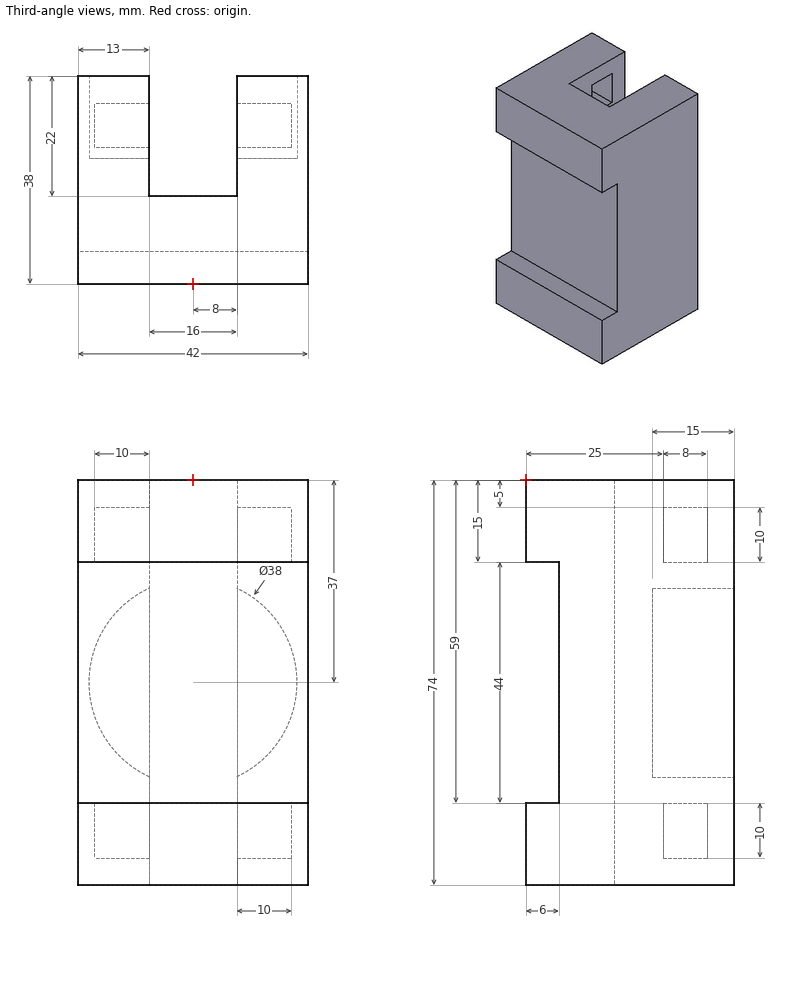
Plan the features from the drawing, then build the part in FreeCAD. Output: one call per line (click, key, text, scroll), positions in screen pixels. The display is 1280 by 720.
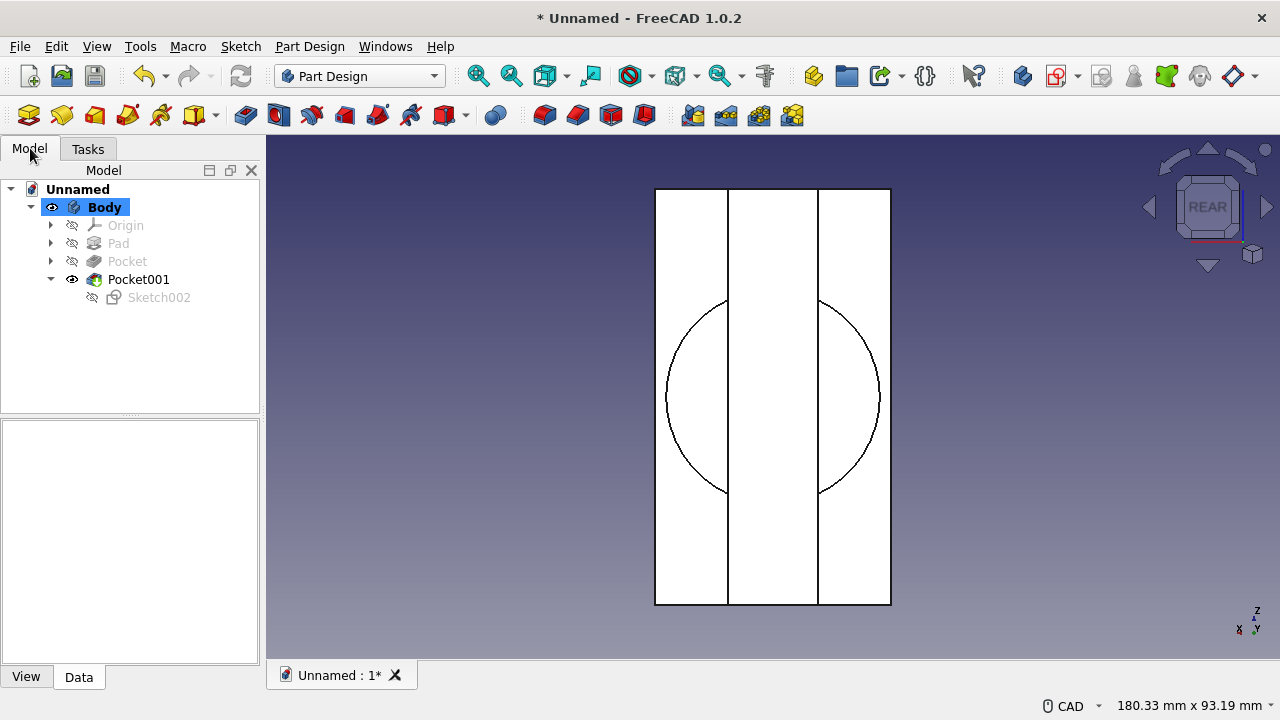
click(51, 225)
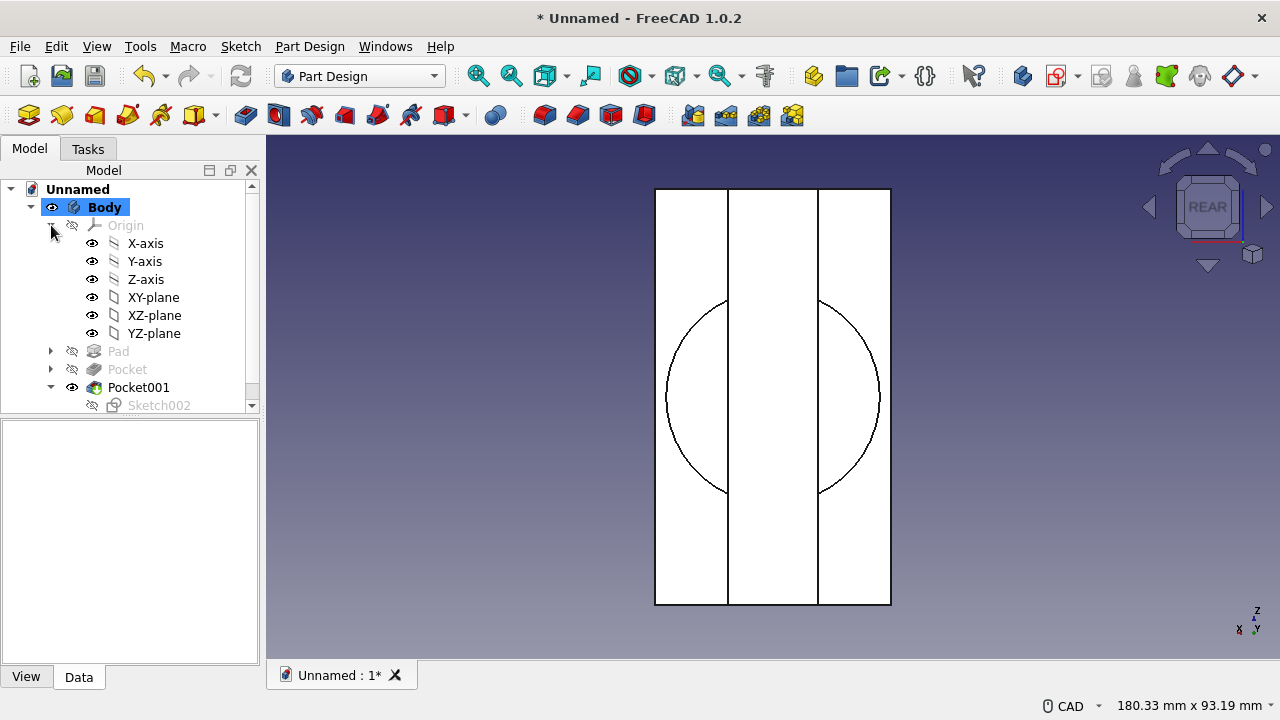
click(137, 333)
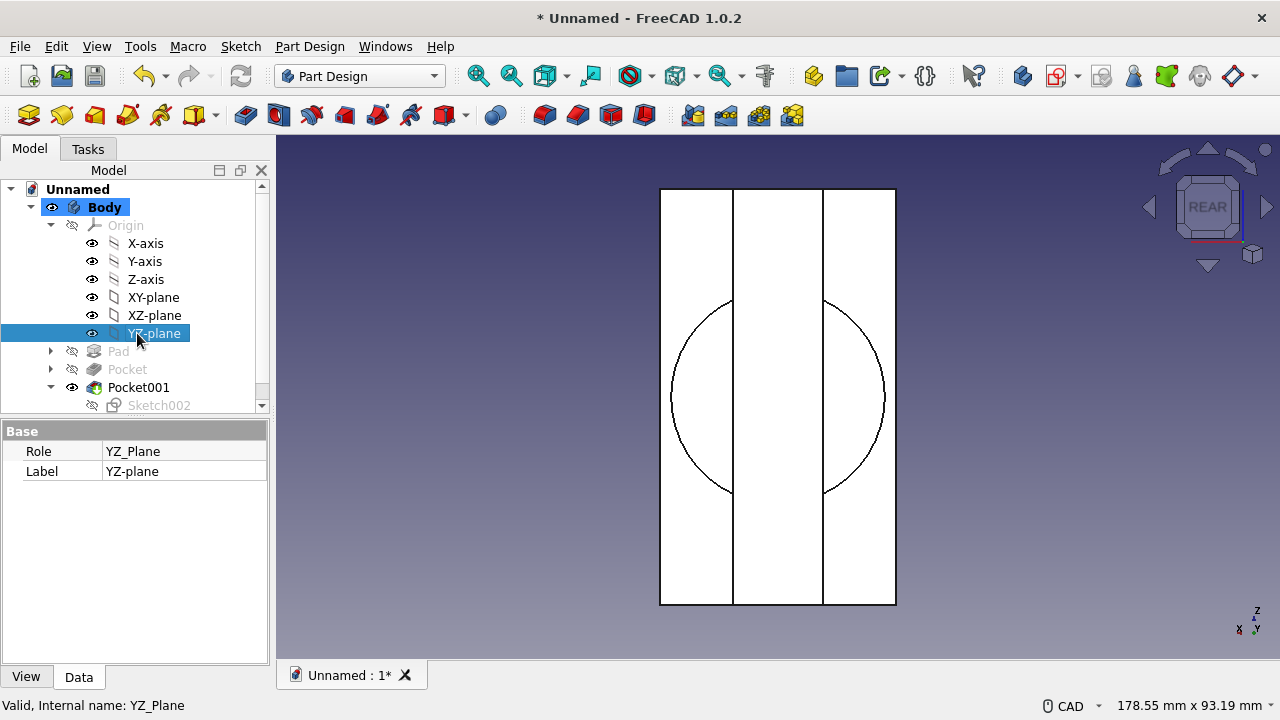
click(1232, 76)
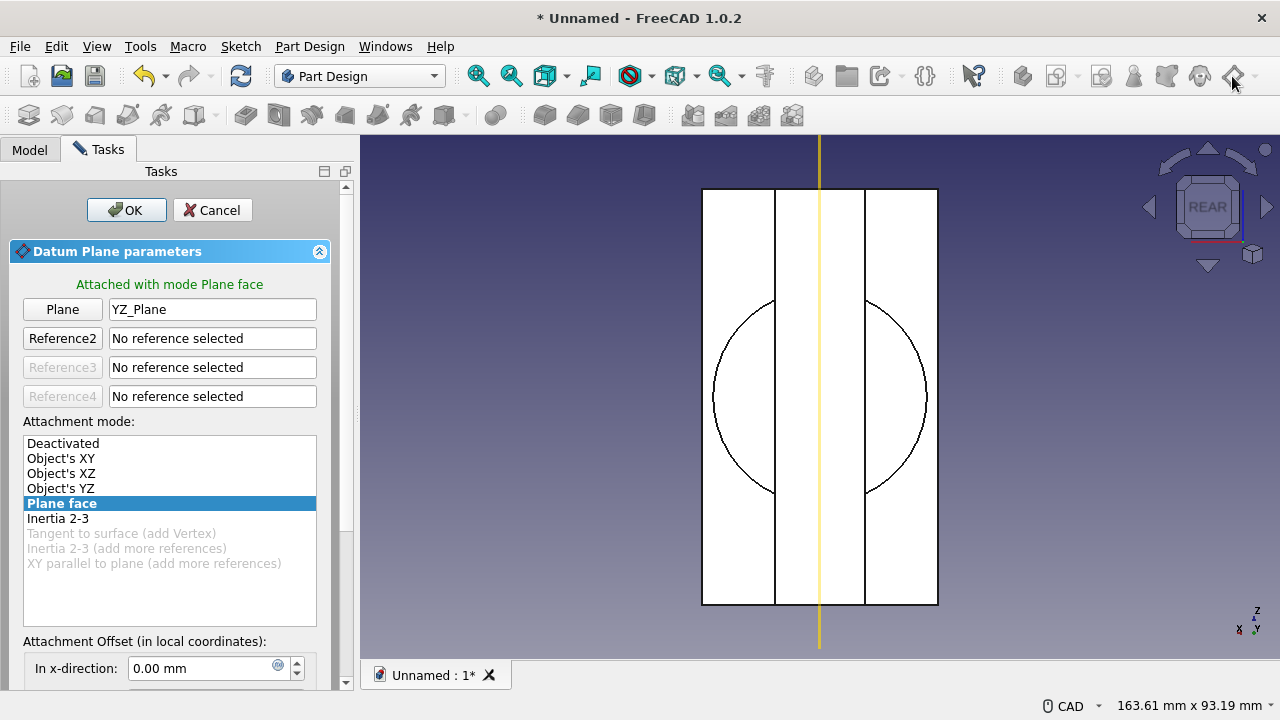
scroll(346, 436, down, 2)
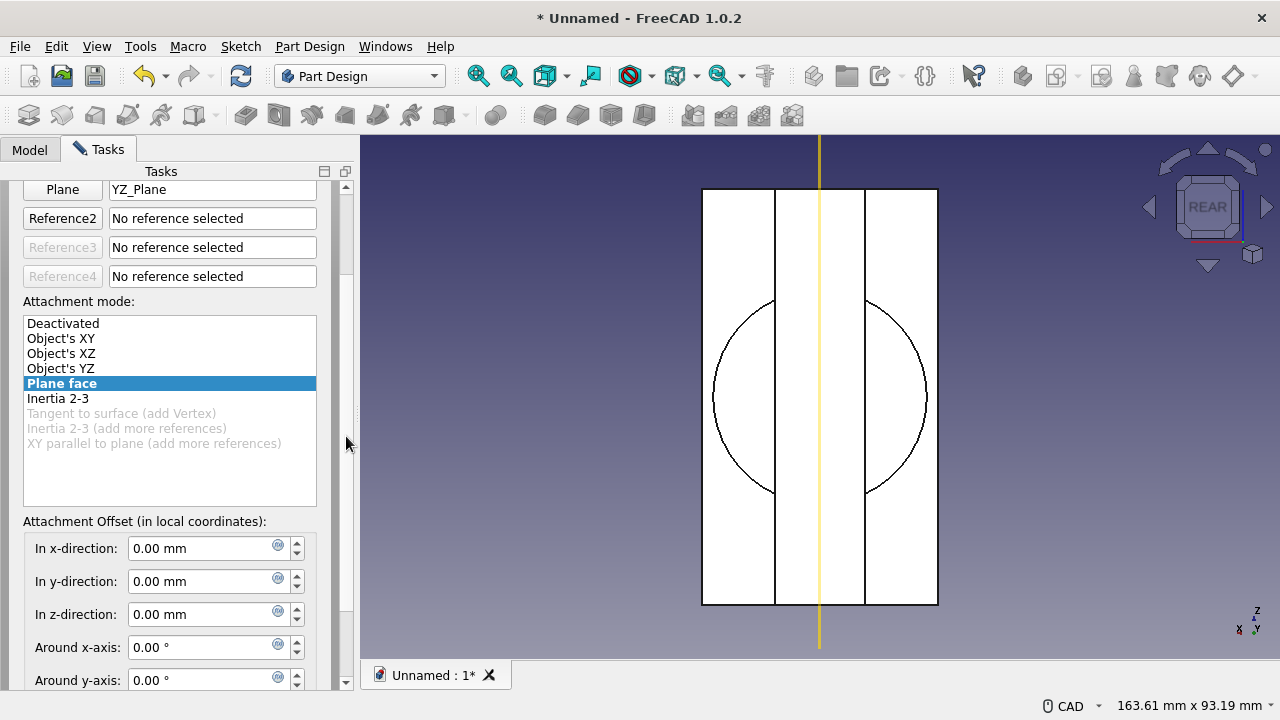
triple_click(210, 614)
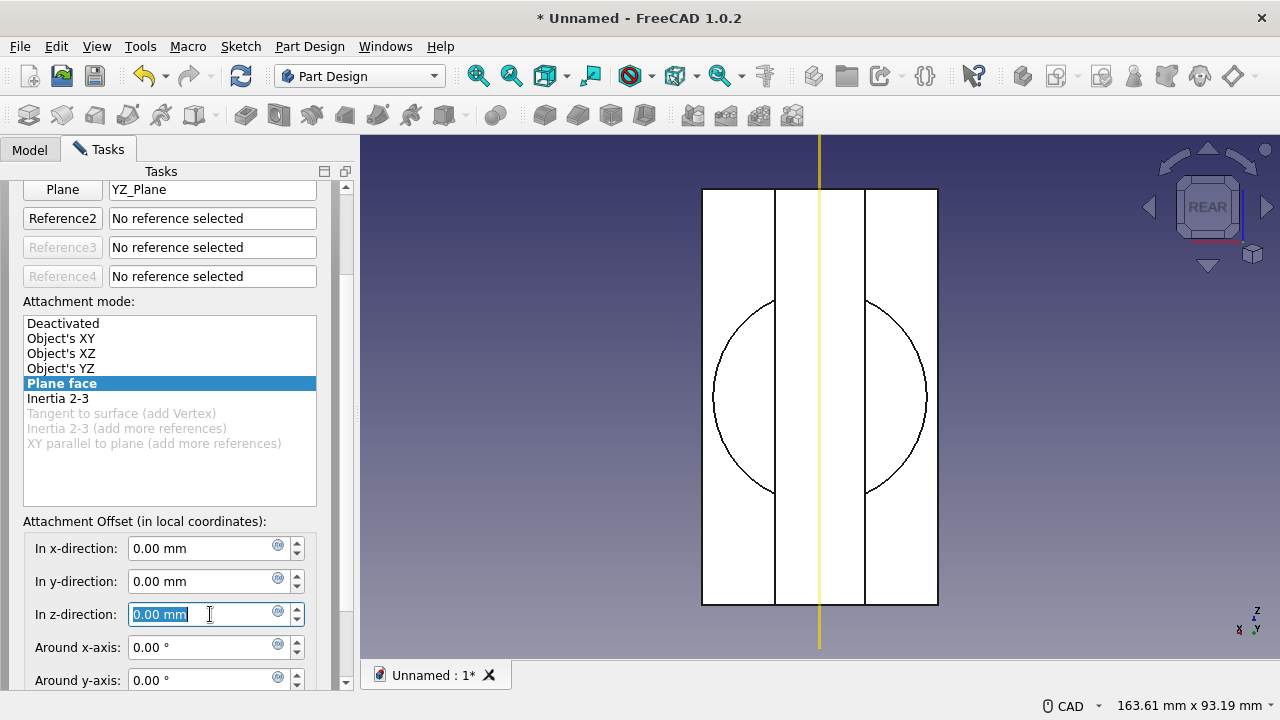
text(-8)
key(Tab)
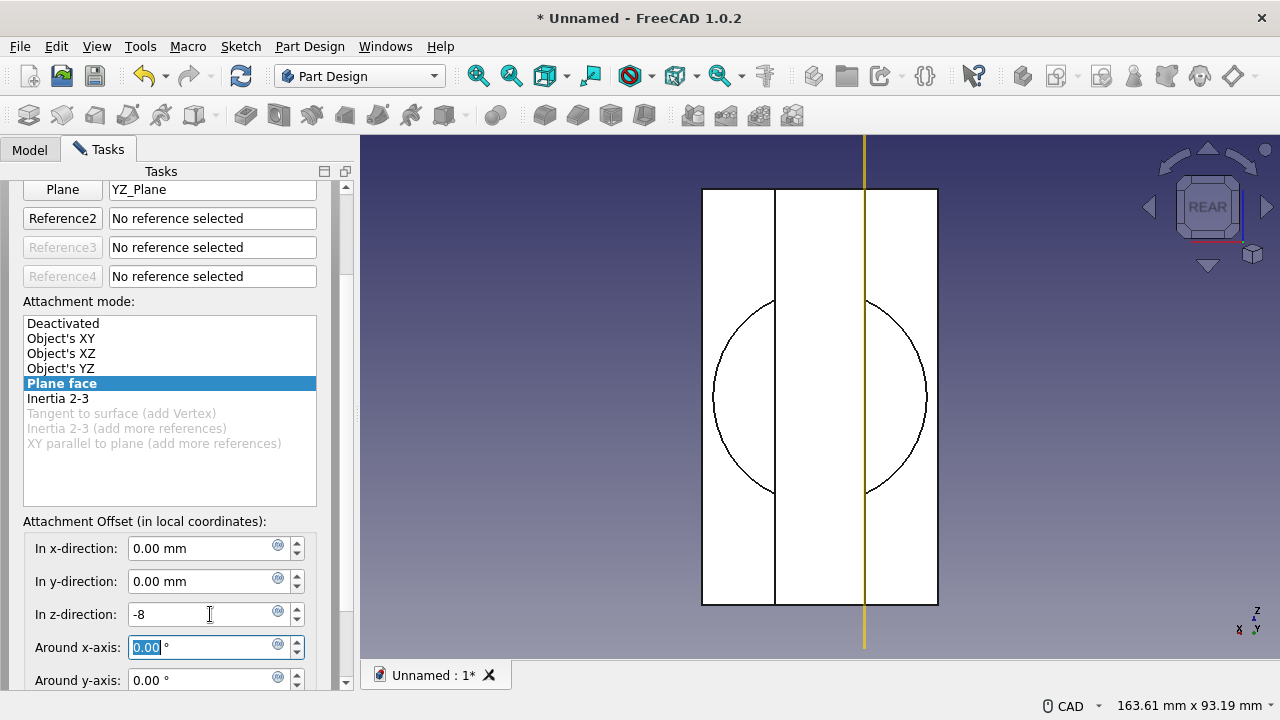
scroll(346, 436, up, 3)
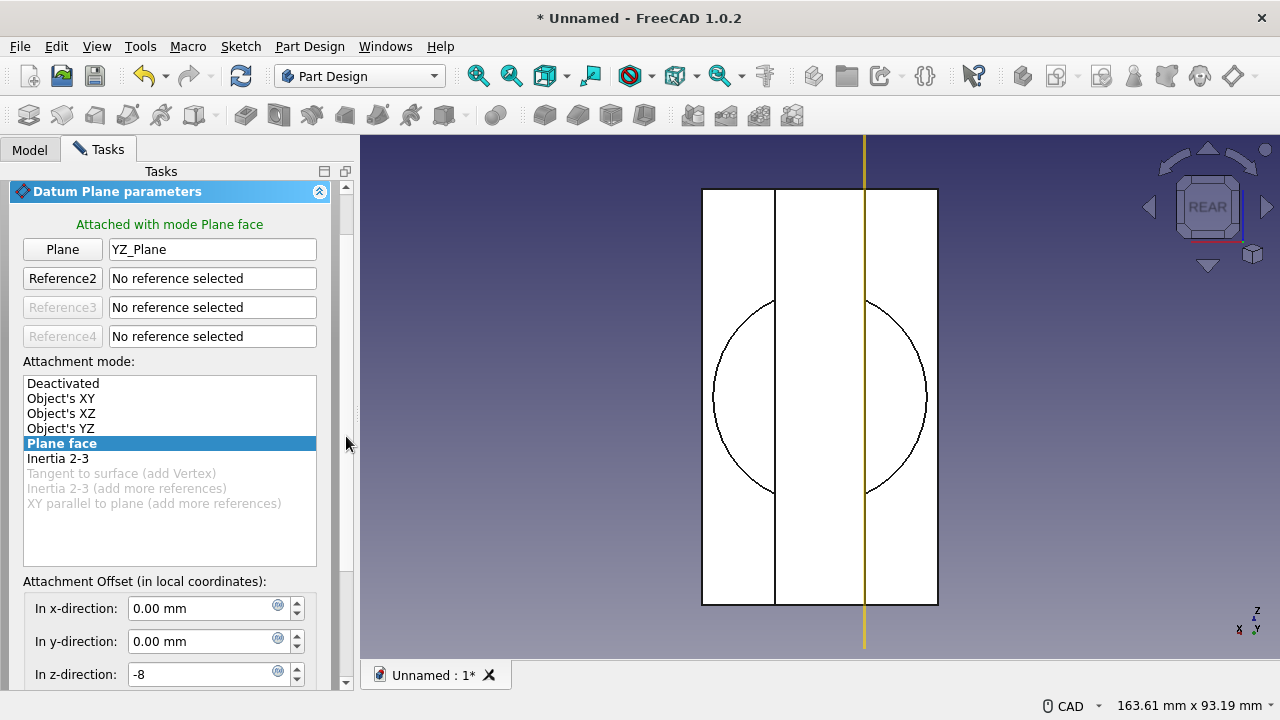
click(127, 210)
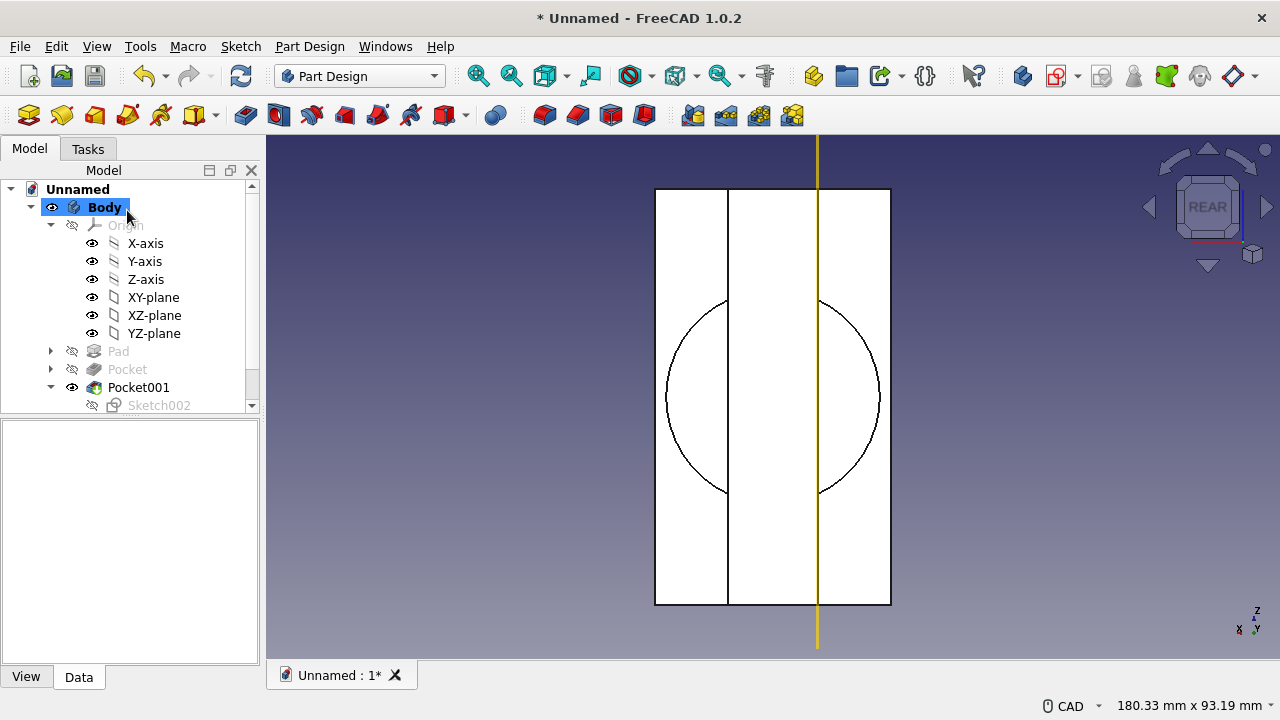
scroll(101, 293, down, 3)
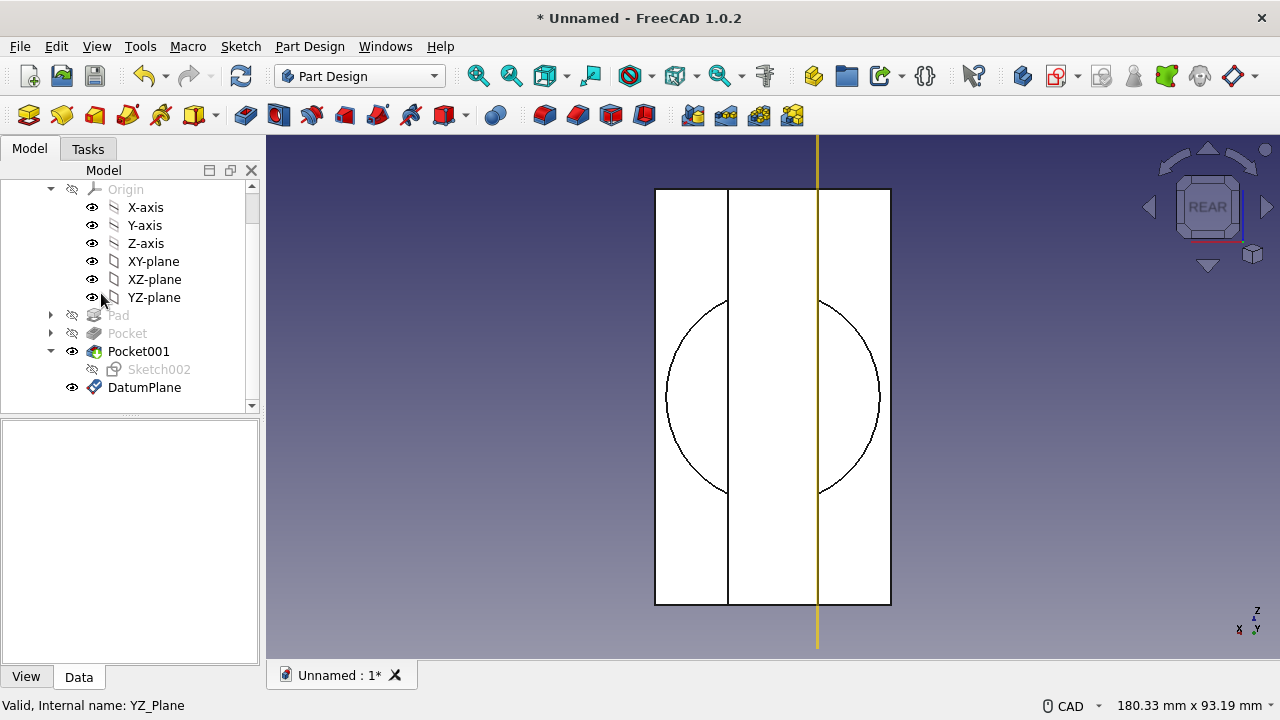
click(117, 387)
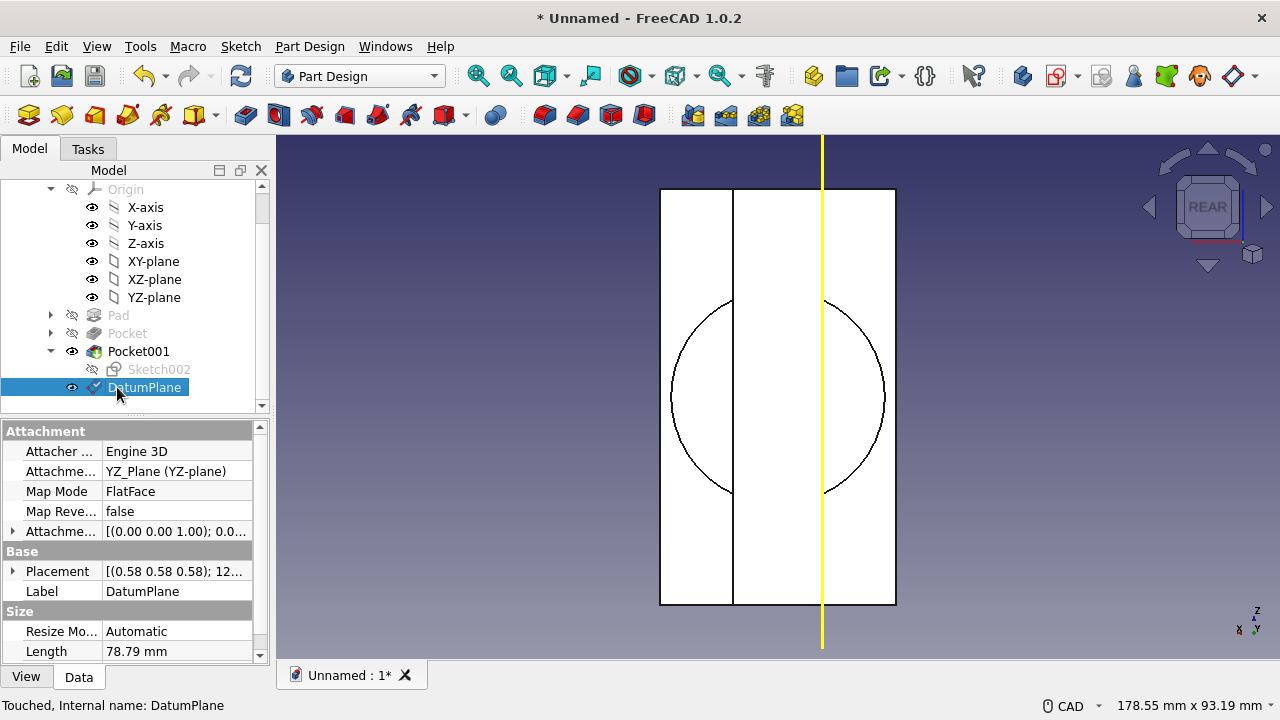
click(1056, 76)